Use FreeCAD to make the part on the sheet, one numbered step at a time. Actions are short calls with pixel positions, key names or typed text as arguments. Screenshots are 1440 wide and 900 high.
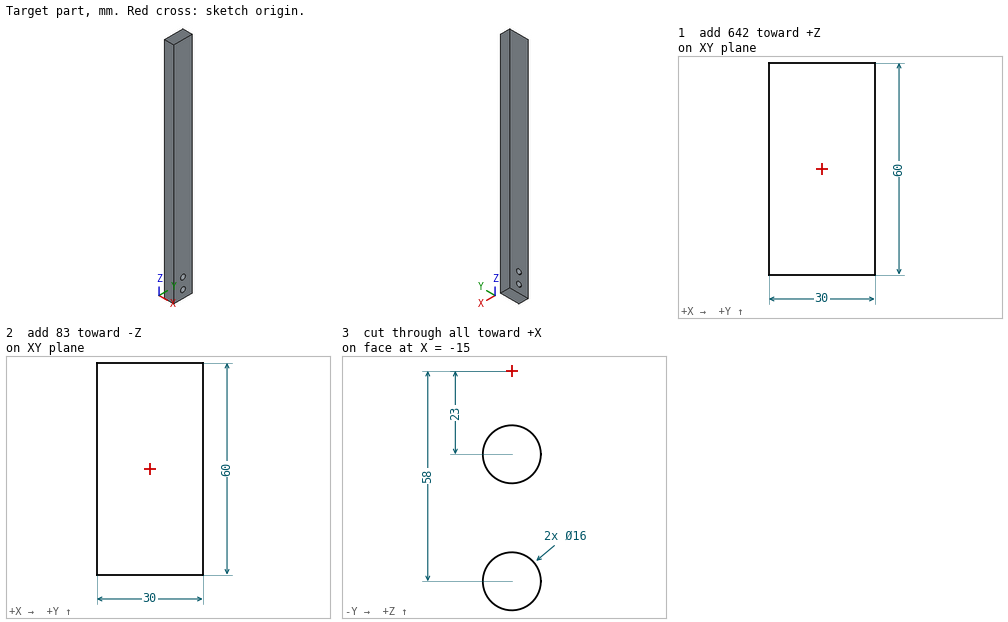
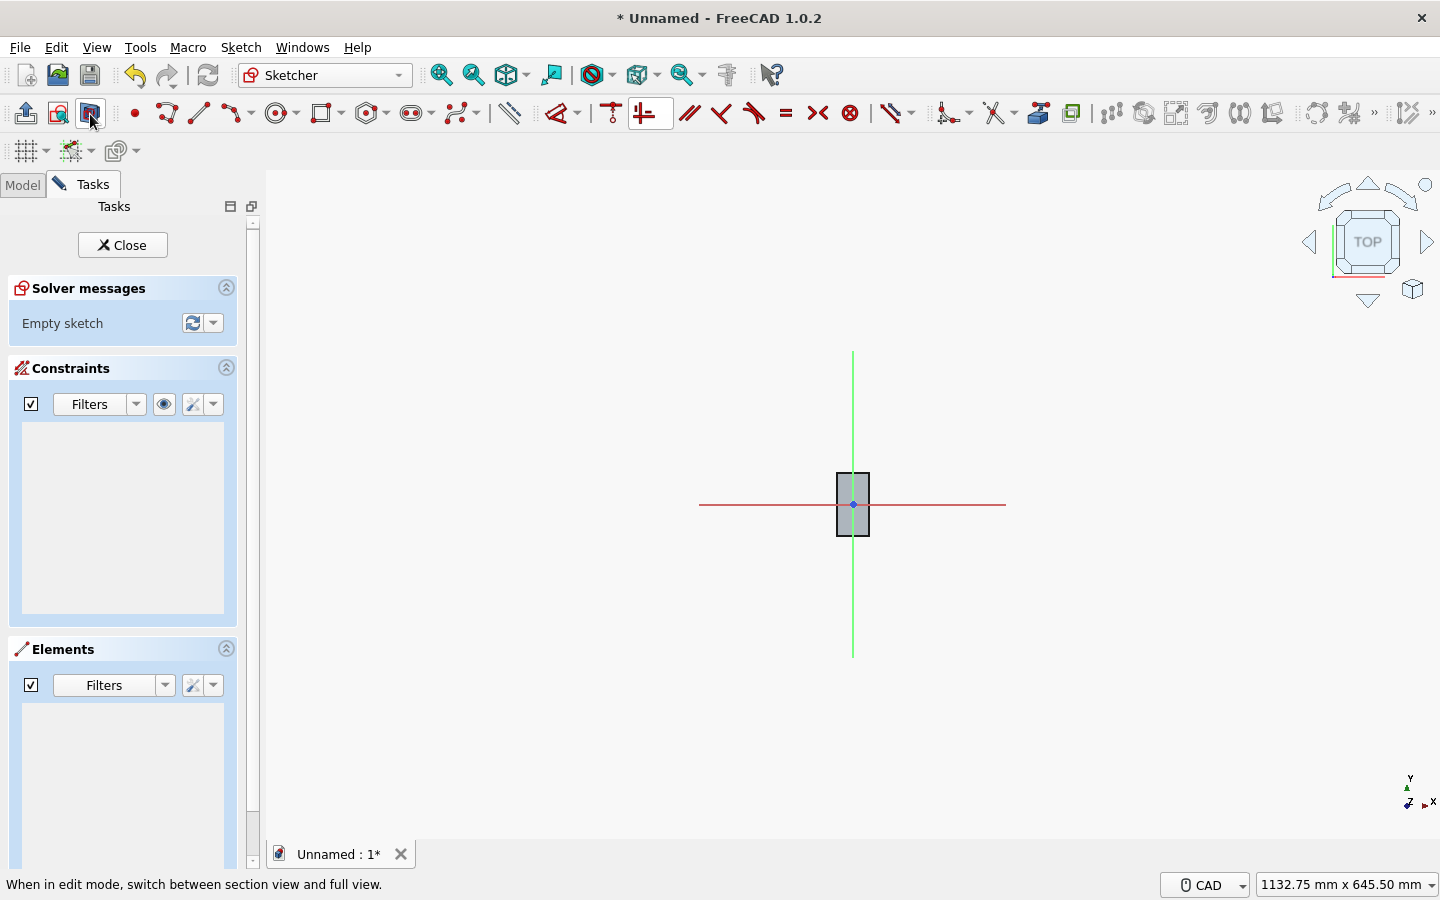
scroll(864, 504, up, 10)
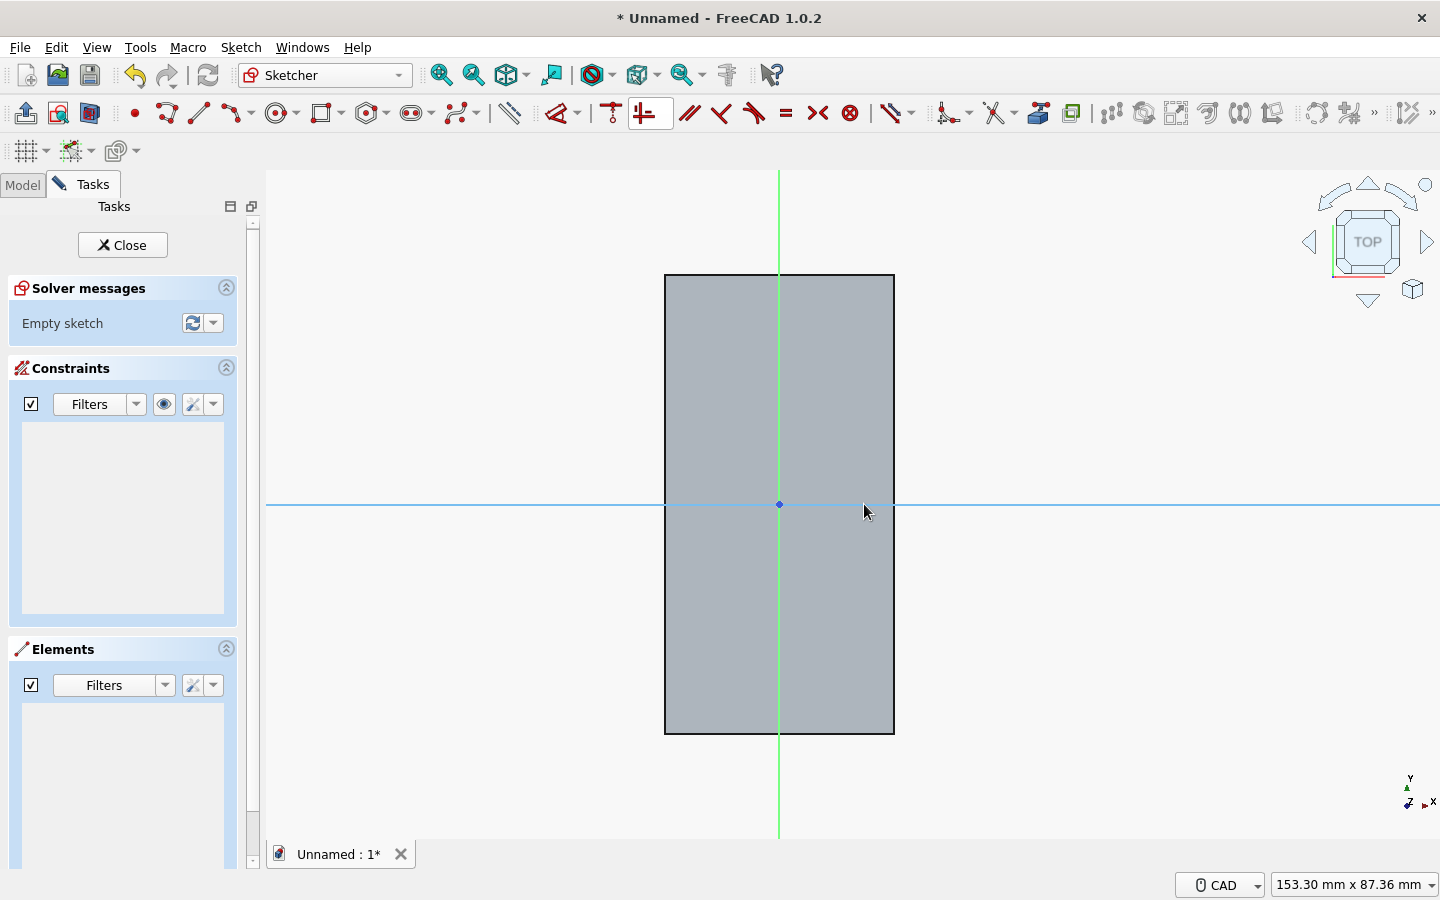
click(344, 114)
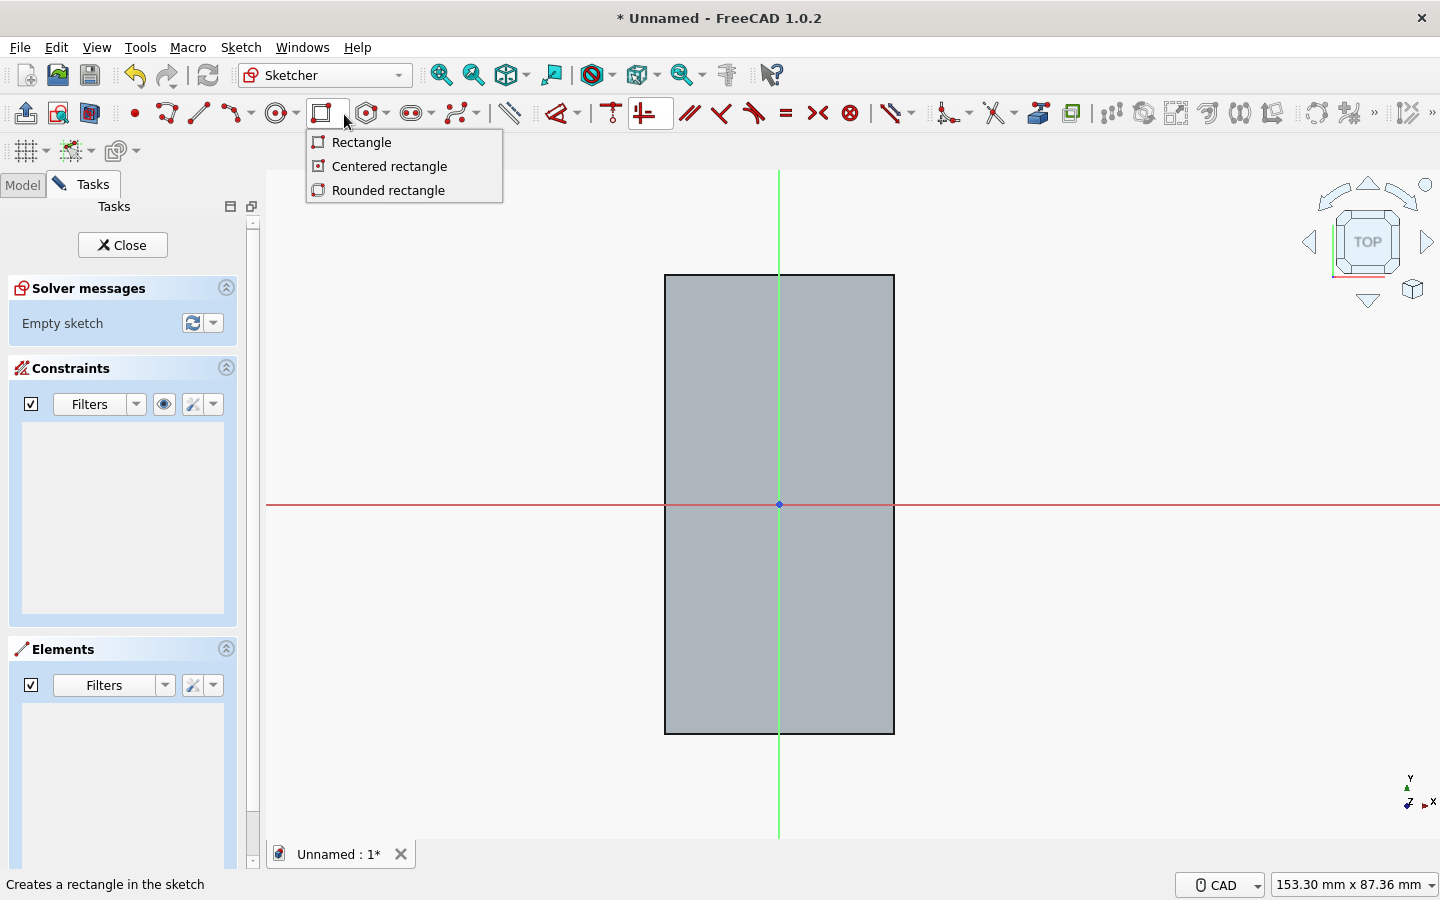
click(404, 166)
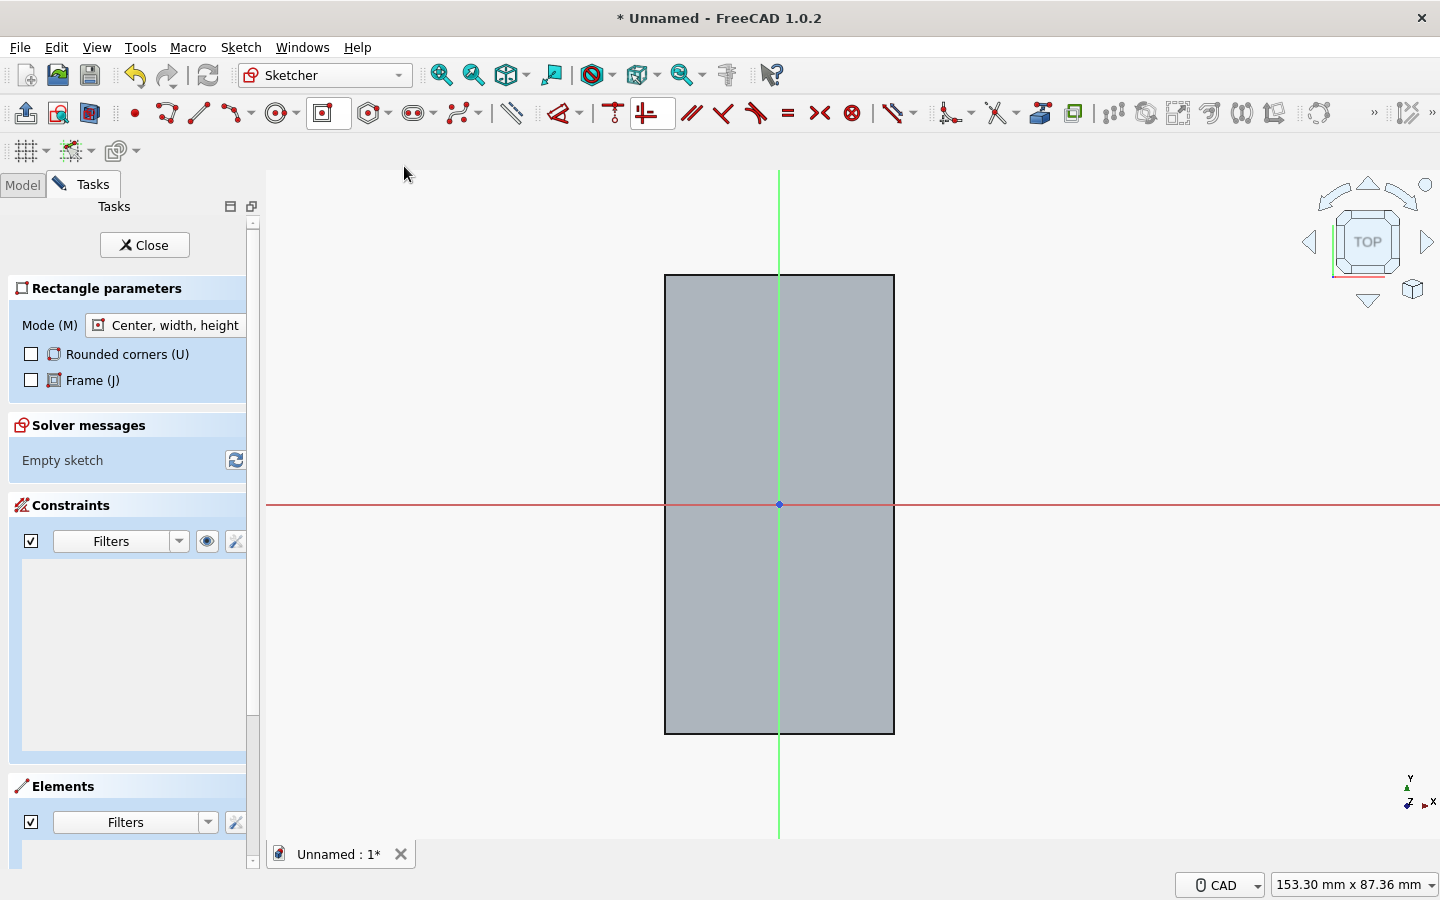
click(779, 504)
move(894, 275)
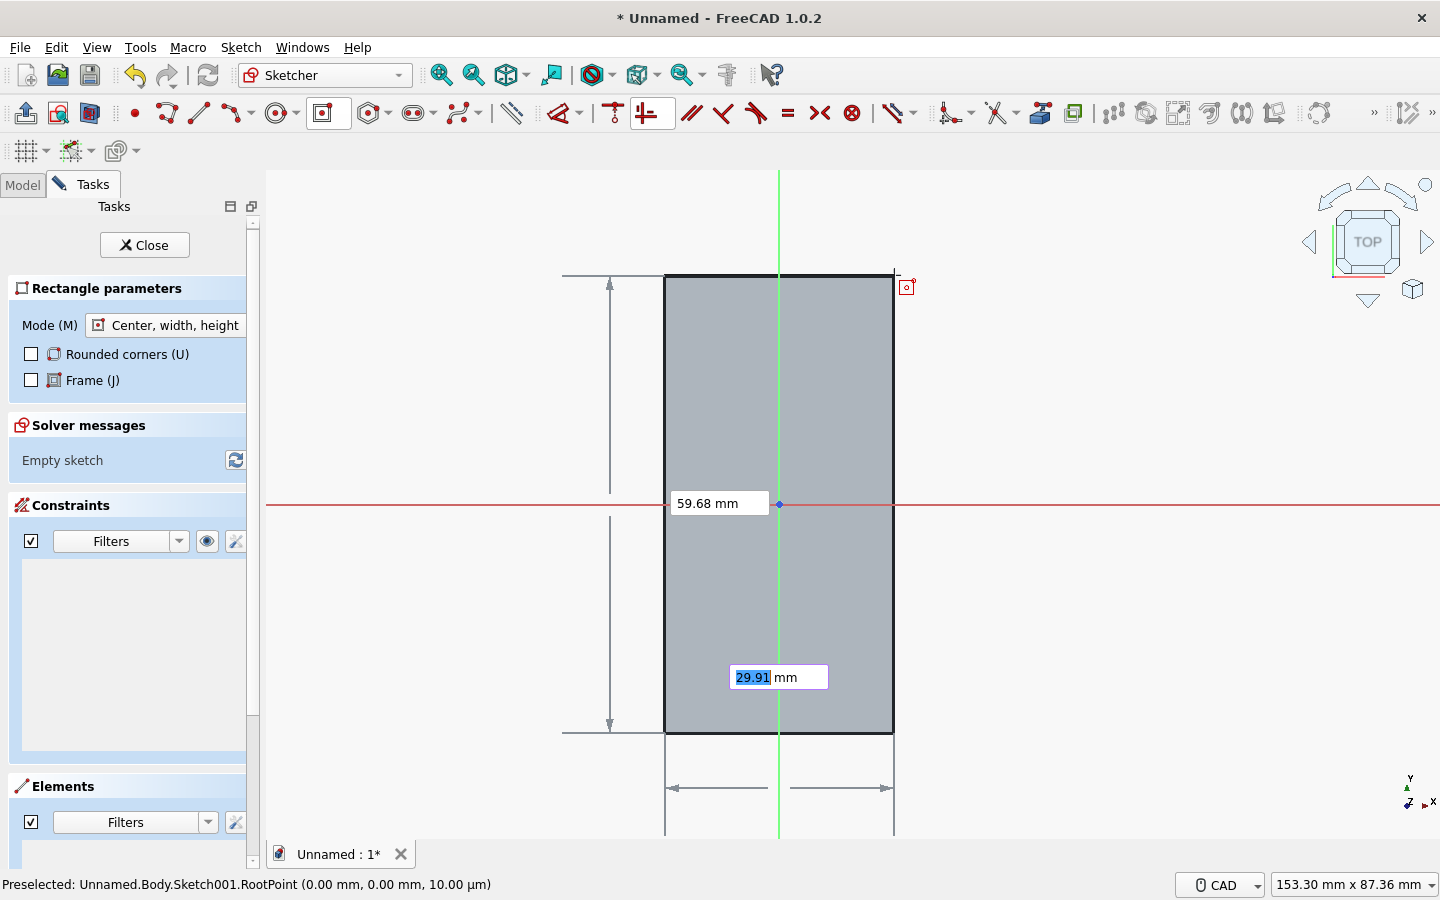
text(30)
key(Tab)
text(60)
key(Return)
key(Escape)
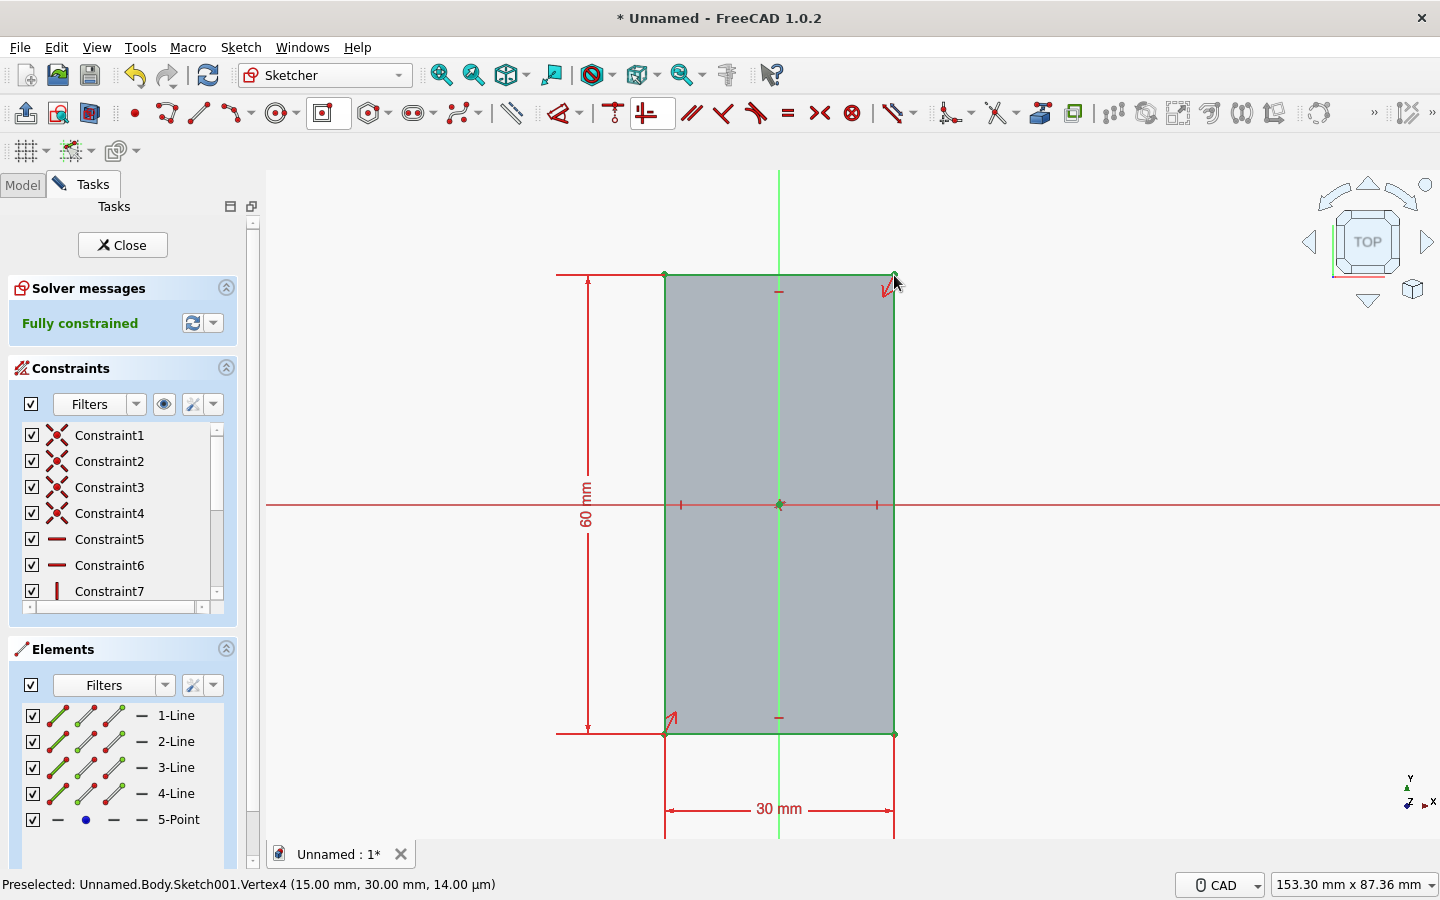
click(123, 245)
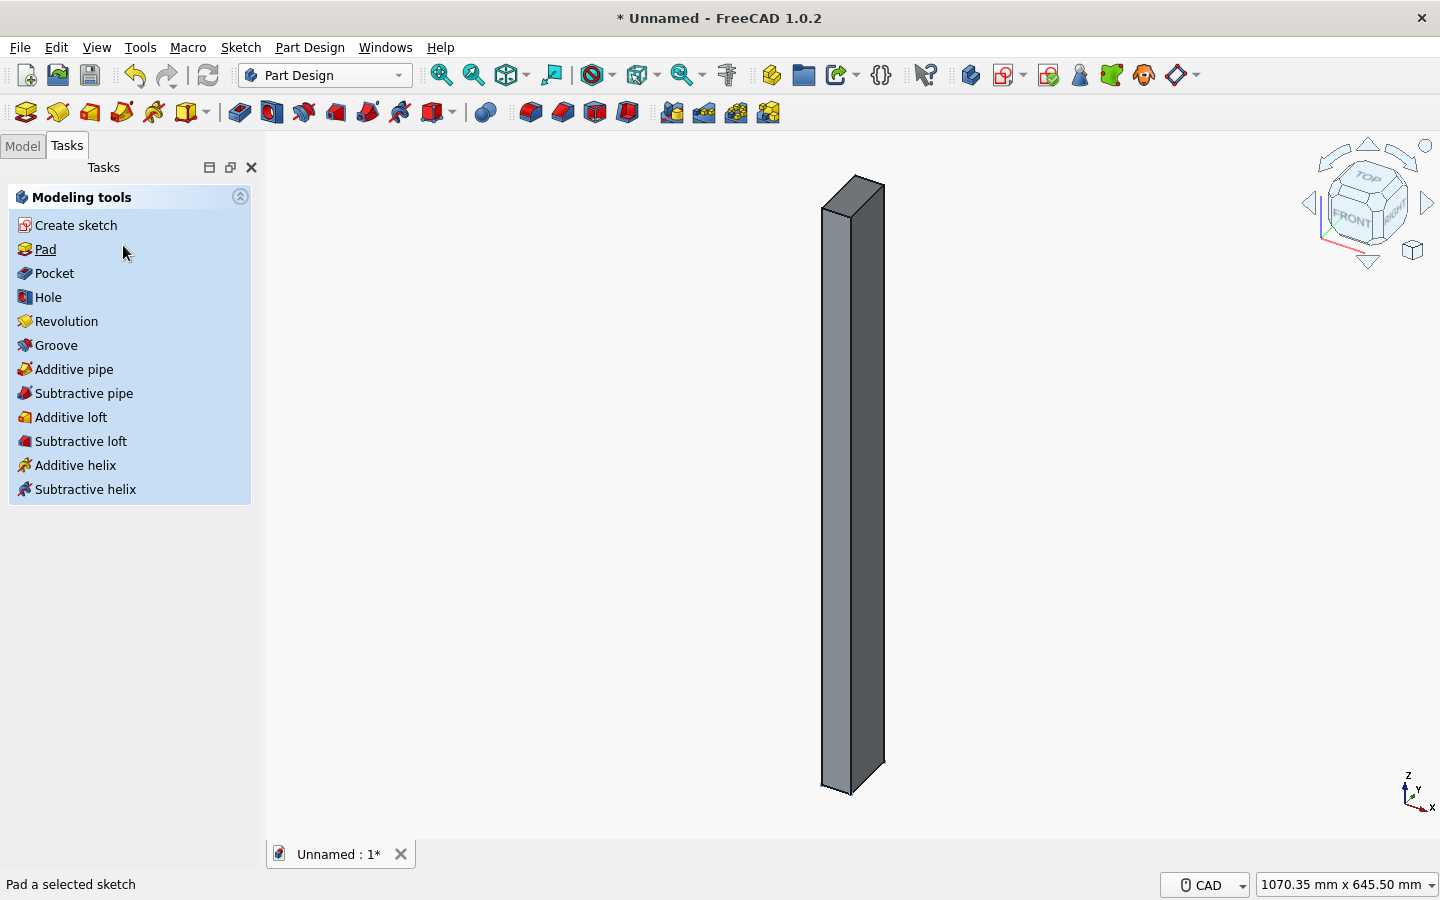
click(26, 112)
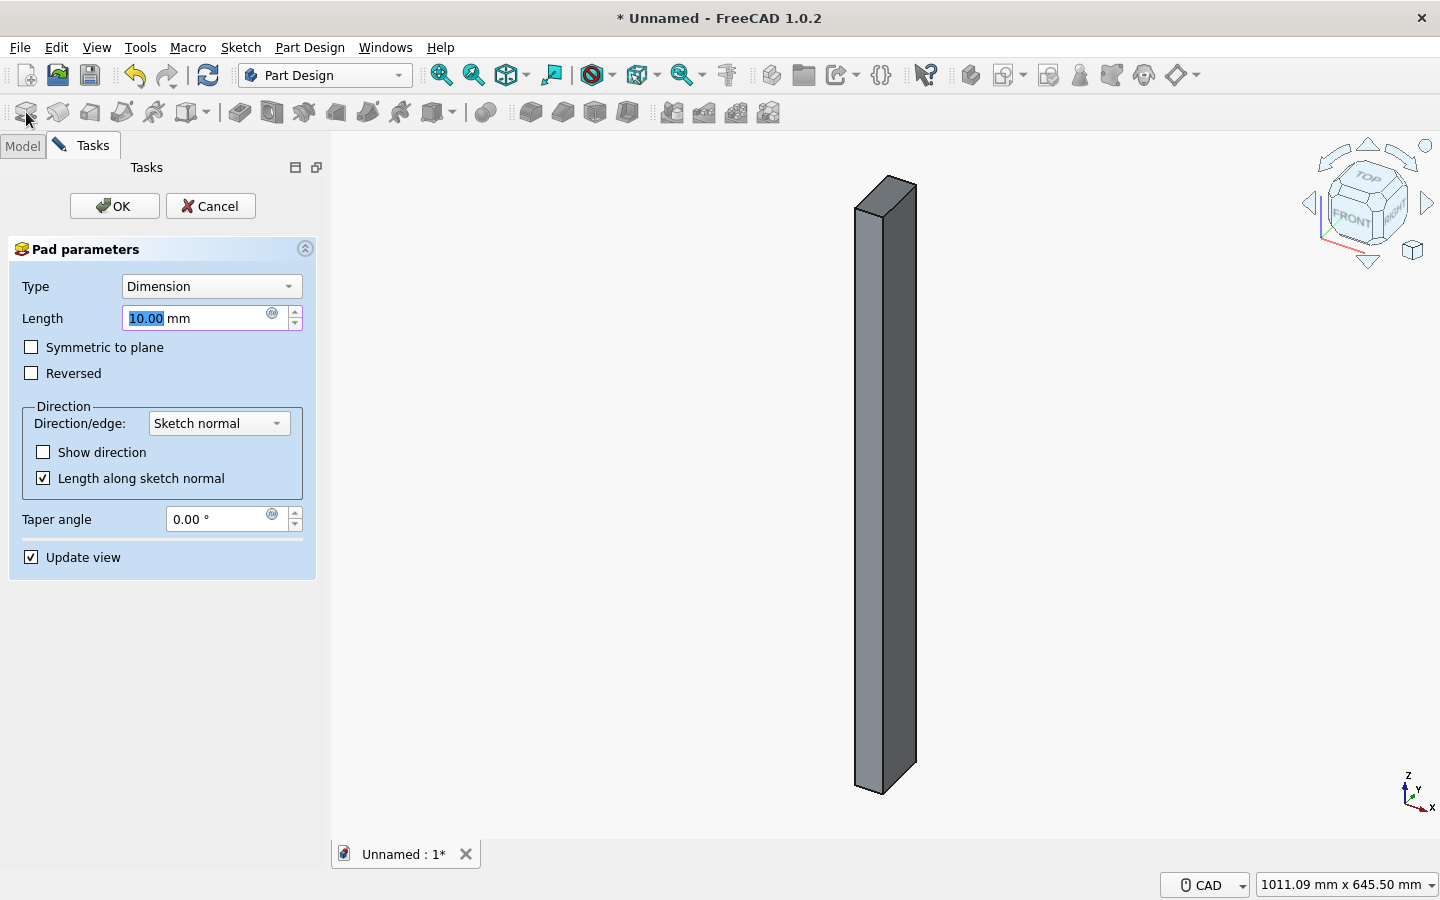
text(83)
key(Tab)